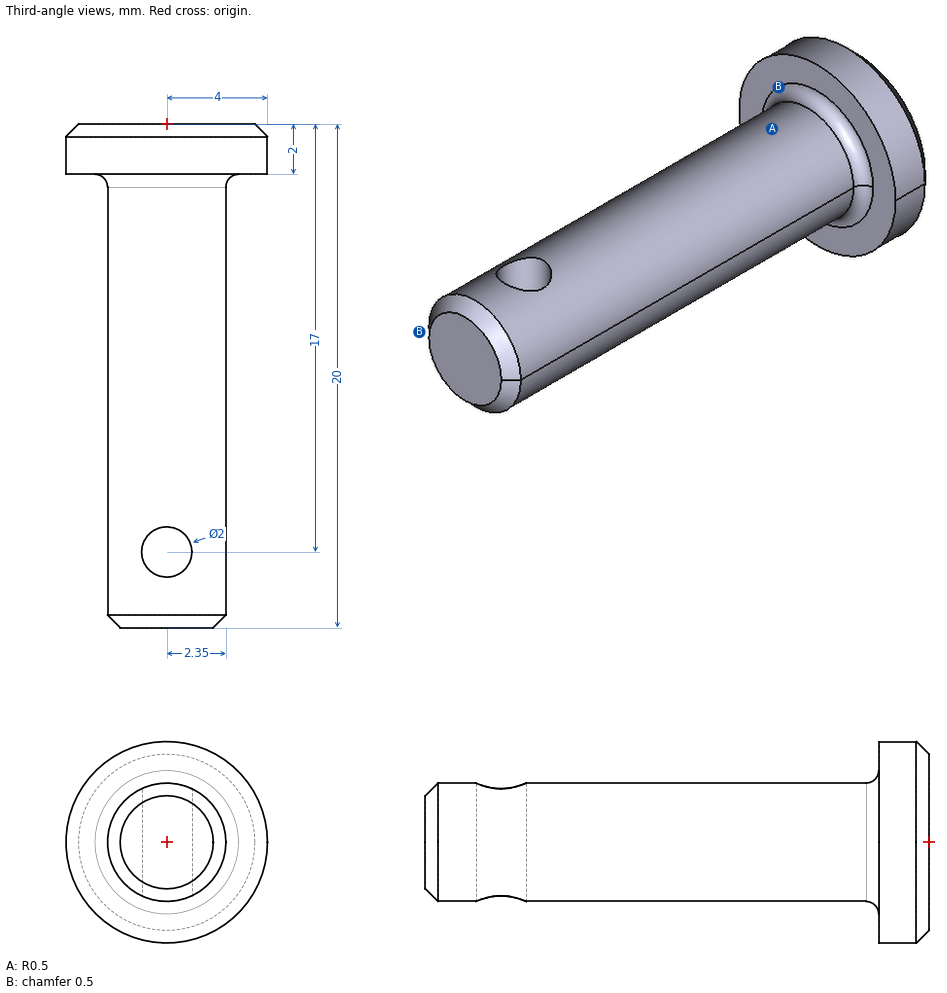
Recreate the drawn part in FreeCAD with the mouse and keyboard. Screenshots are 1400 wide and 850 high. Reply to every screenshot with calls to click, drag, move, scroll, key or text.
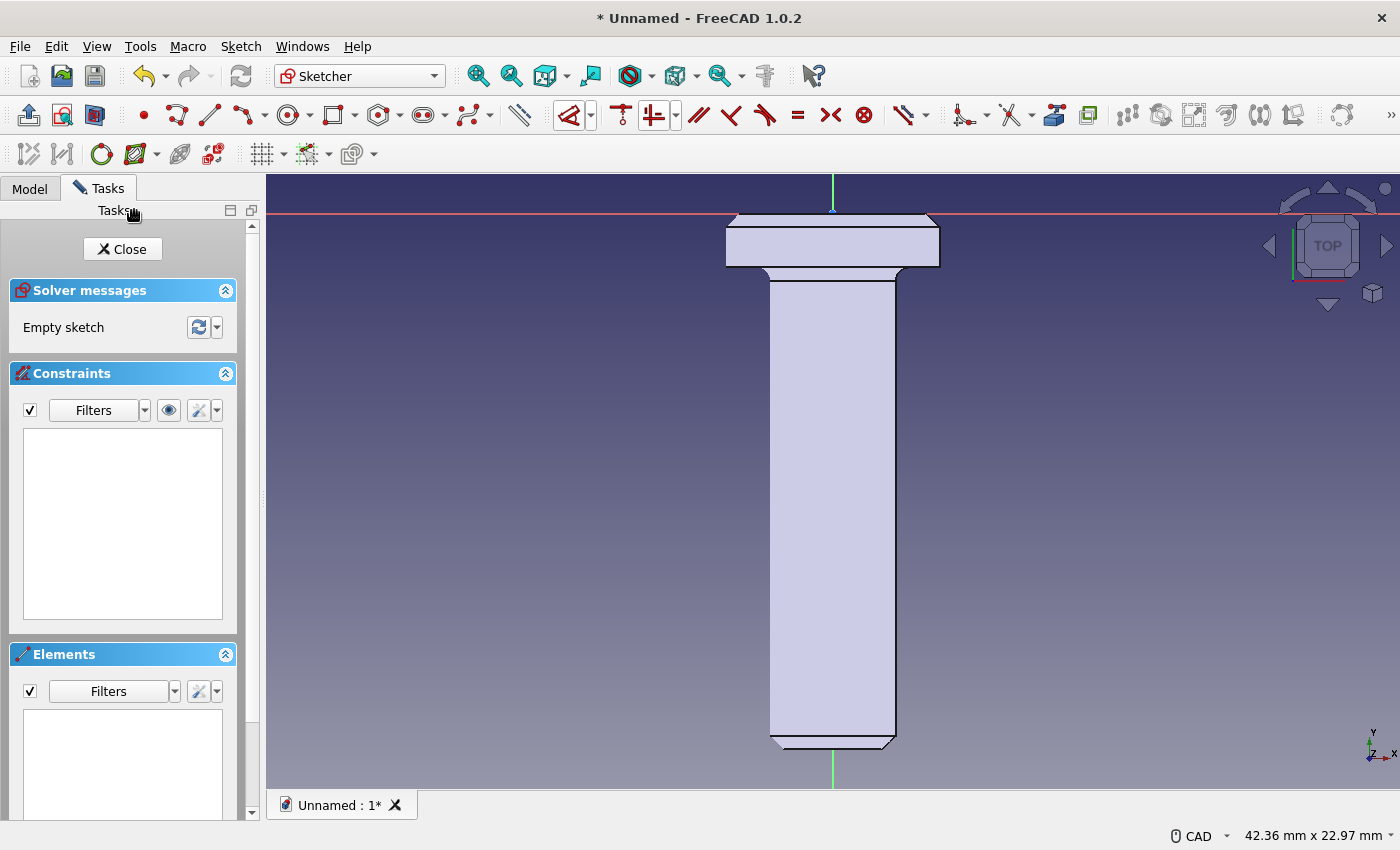
click(95, 116)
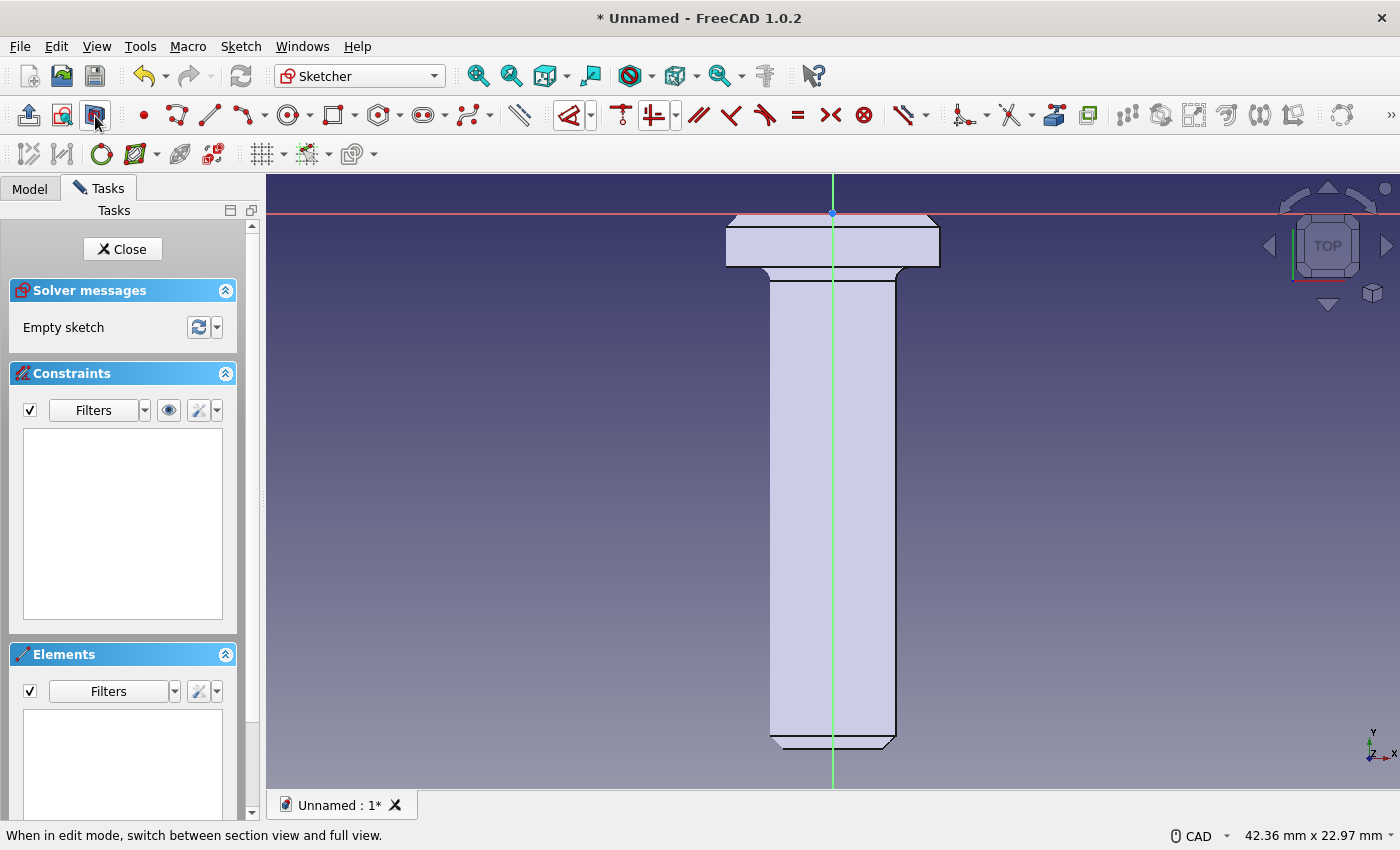
scroll(844, 698, up, 10)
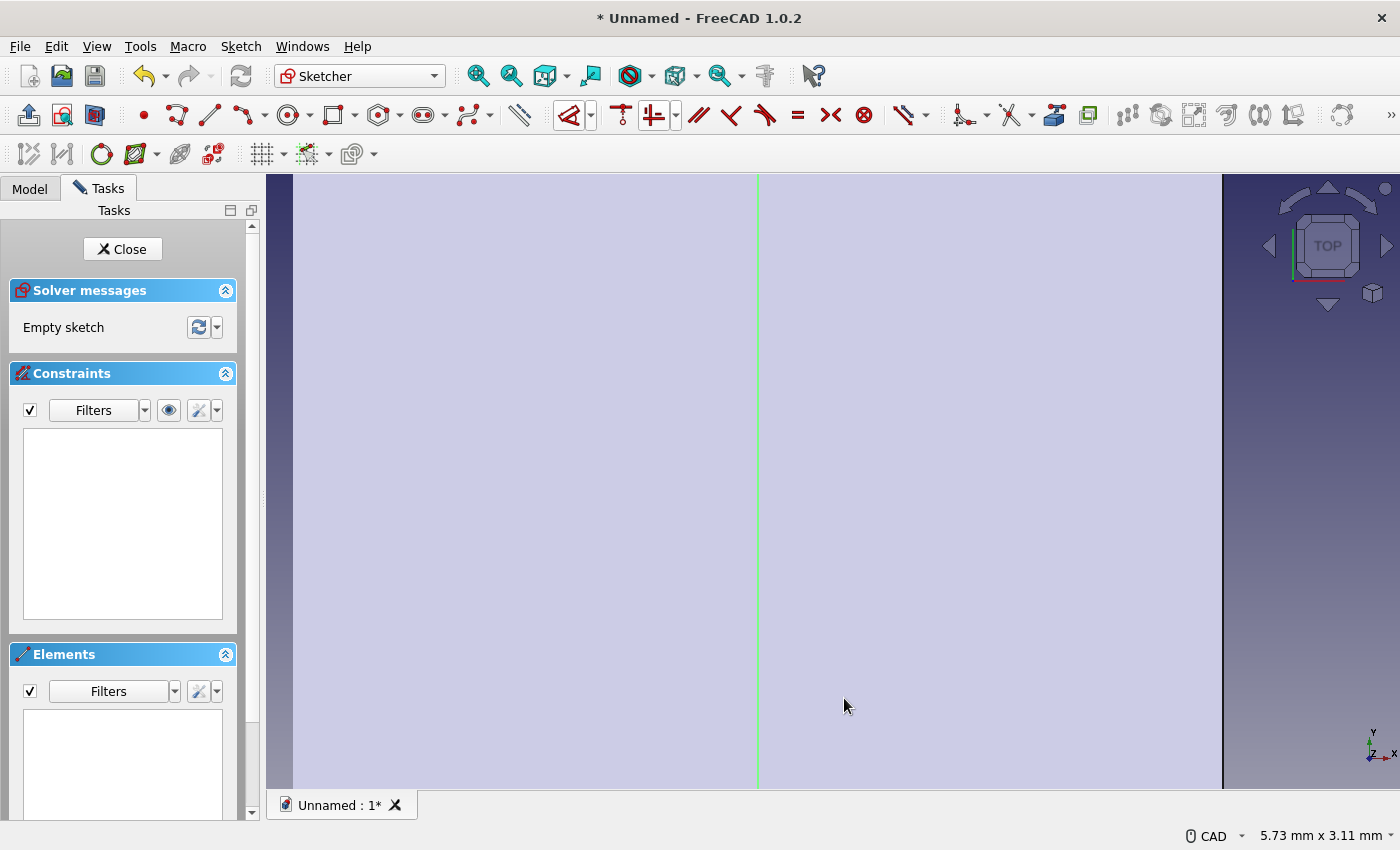
key(g)
key(c)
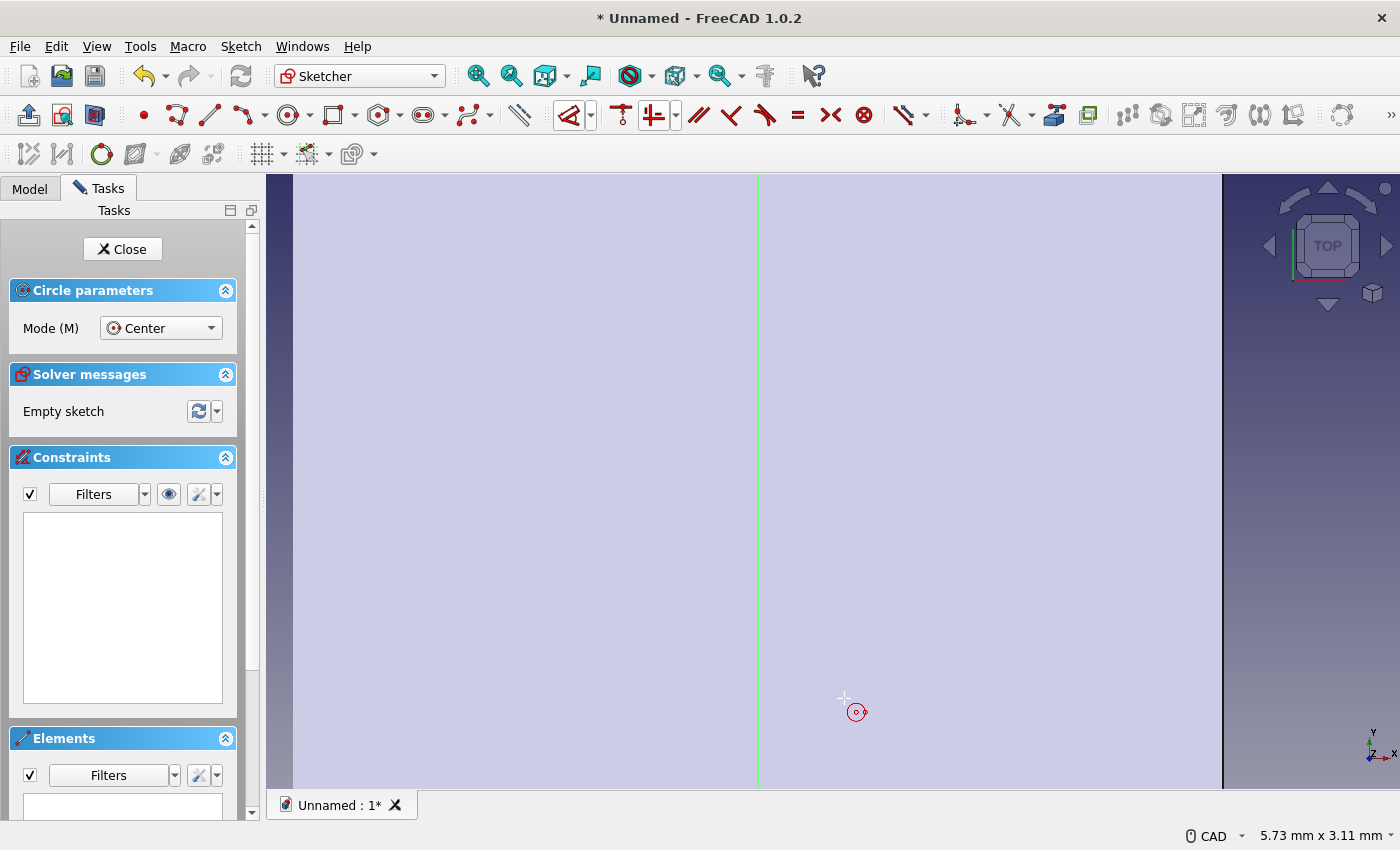
click(758, 478)
click(898, 338)
key(Escape)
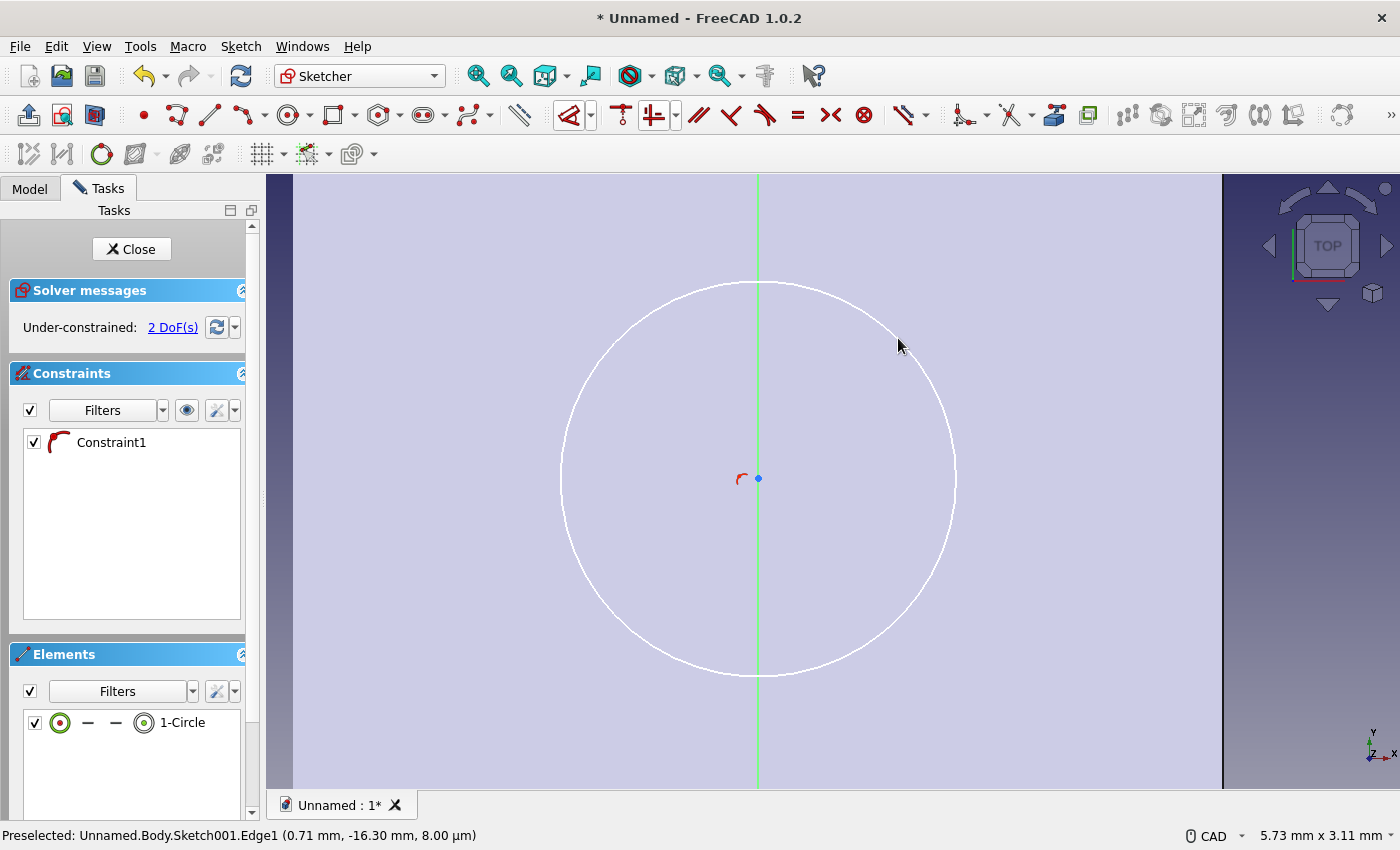
key(d)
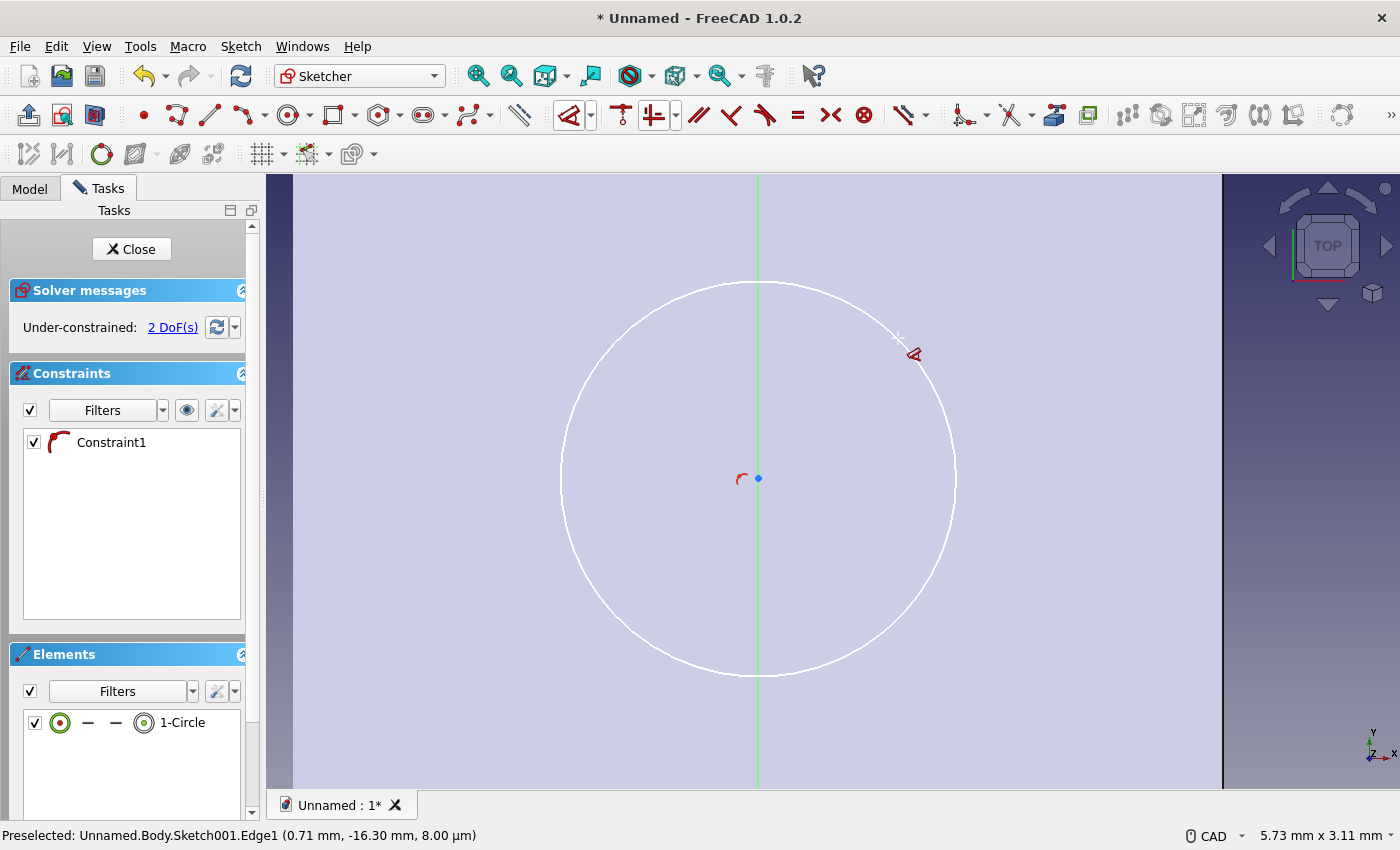
click(898, 339)
click(921, 316)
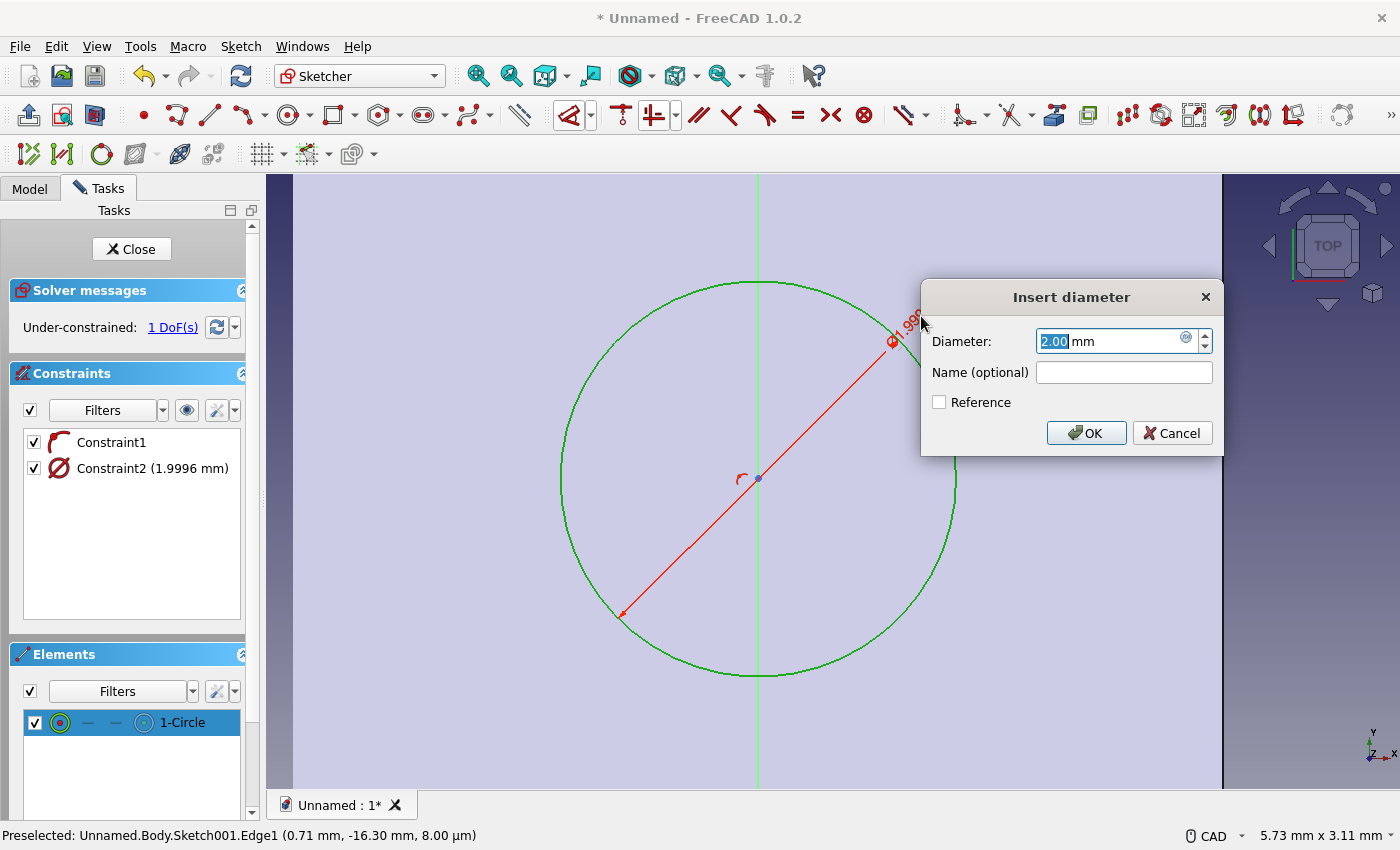
text(2)
key(Return)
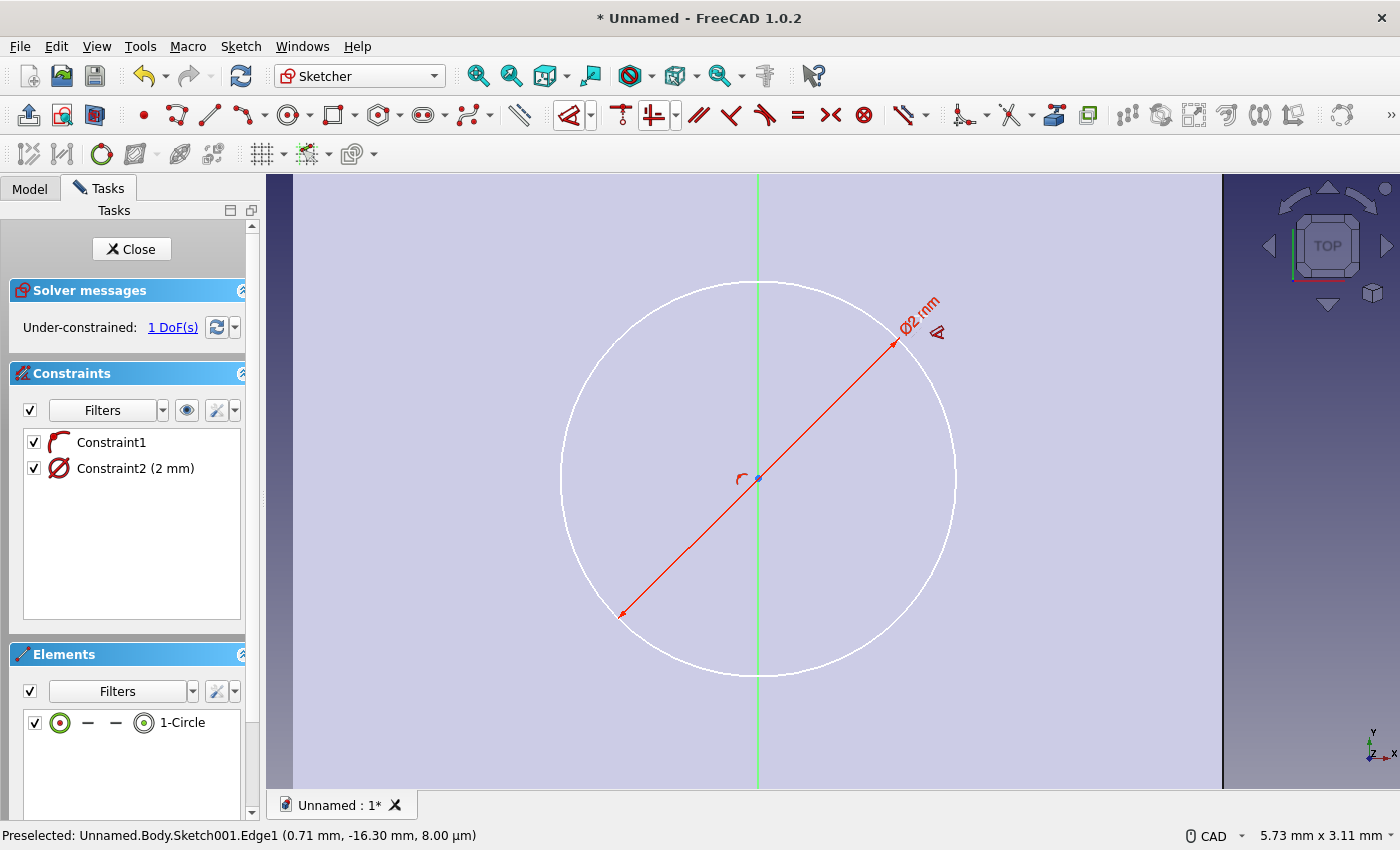
click(758, 479)
click(792, 340)